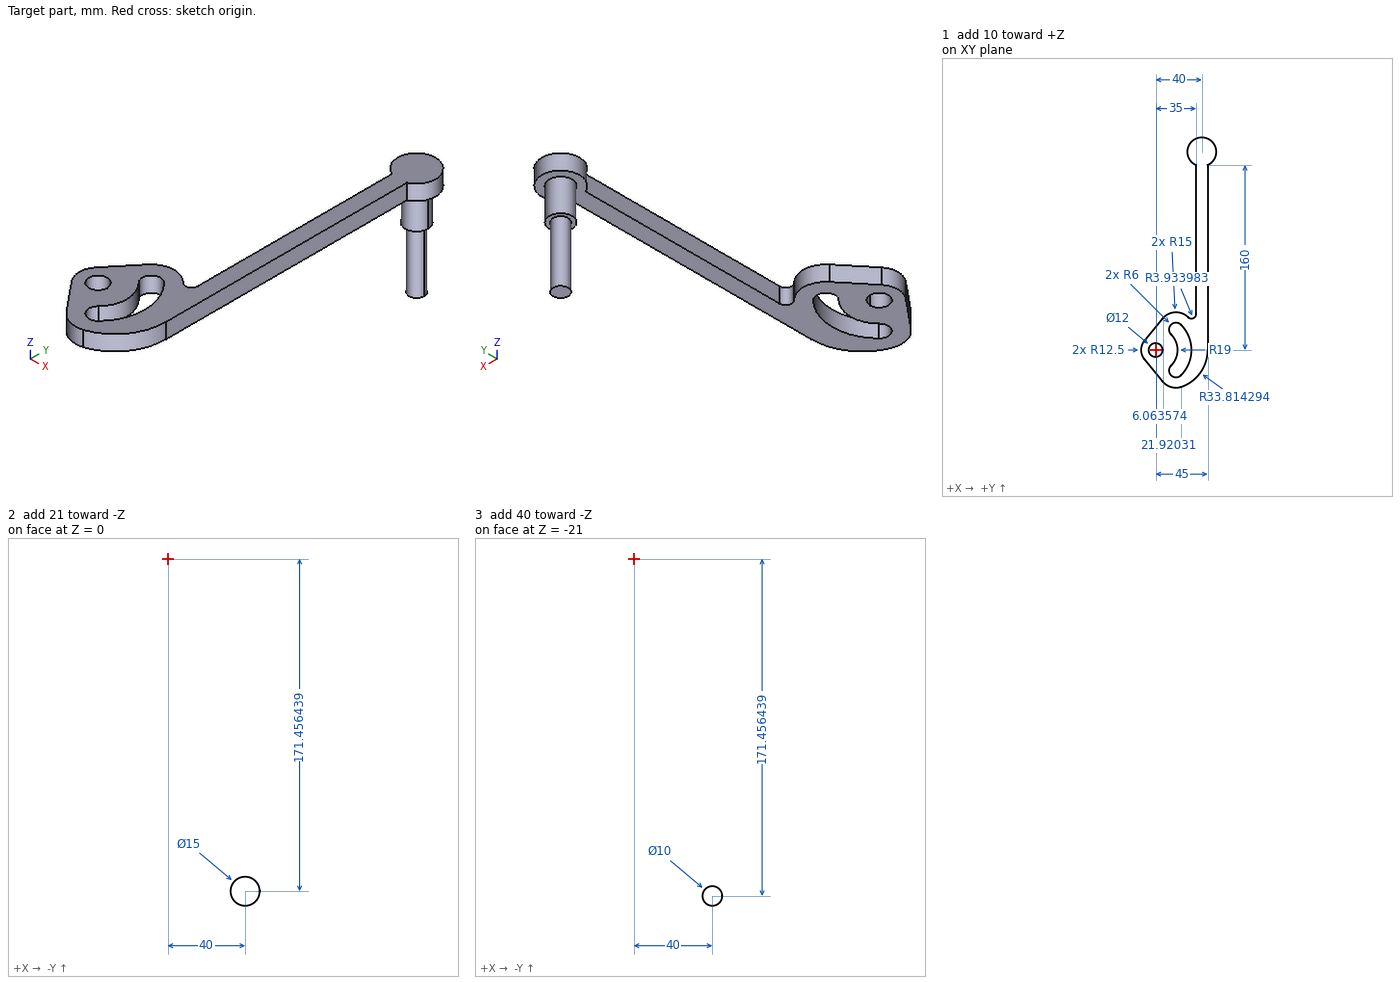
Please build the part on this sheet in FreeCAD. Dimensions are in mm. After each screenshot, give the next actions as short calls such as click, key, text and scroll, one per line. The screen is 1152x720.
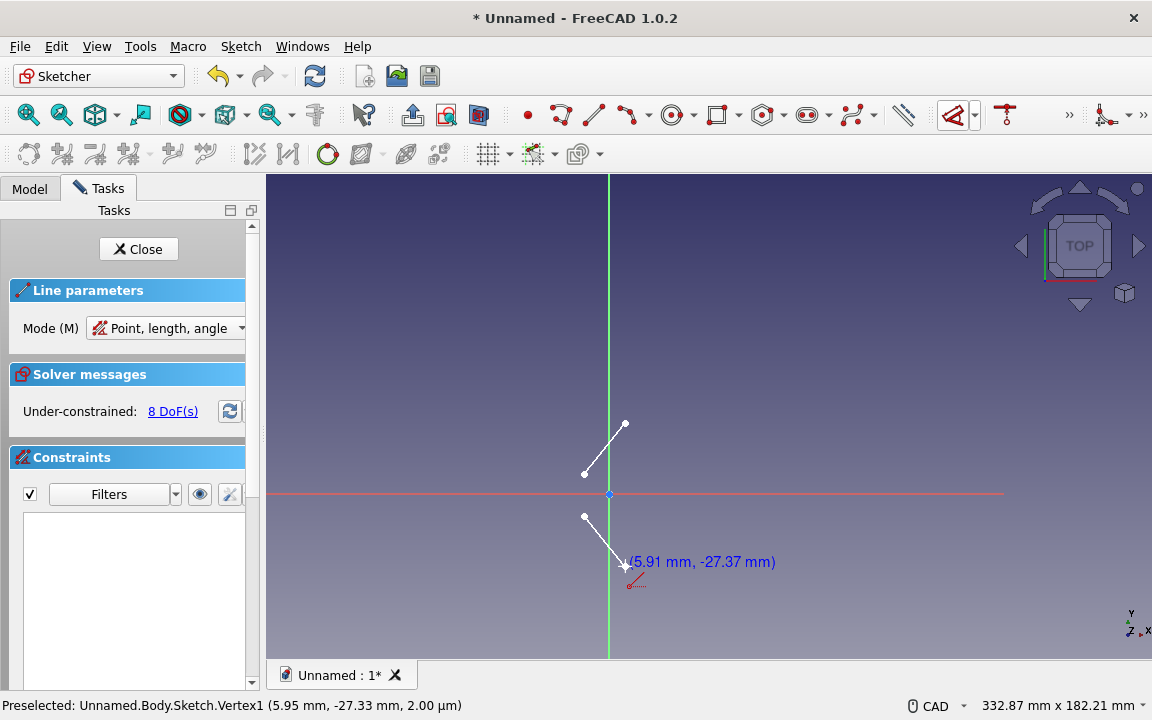
click(729, 494)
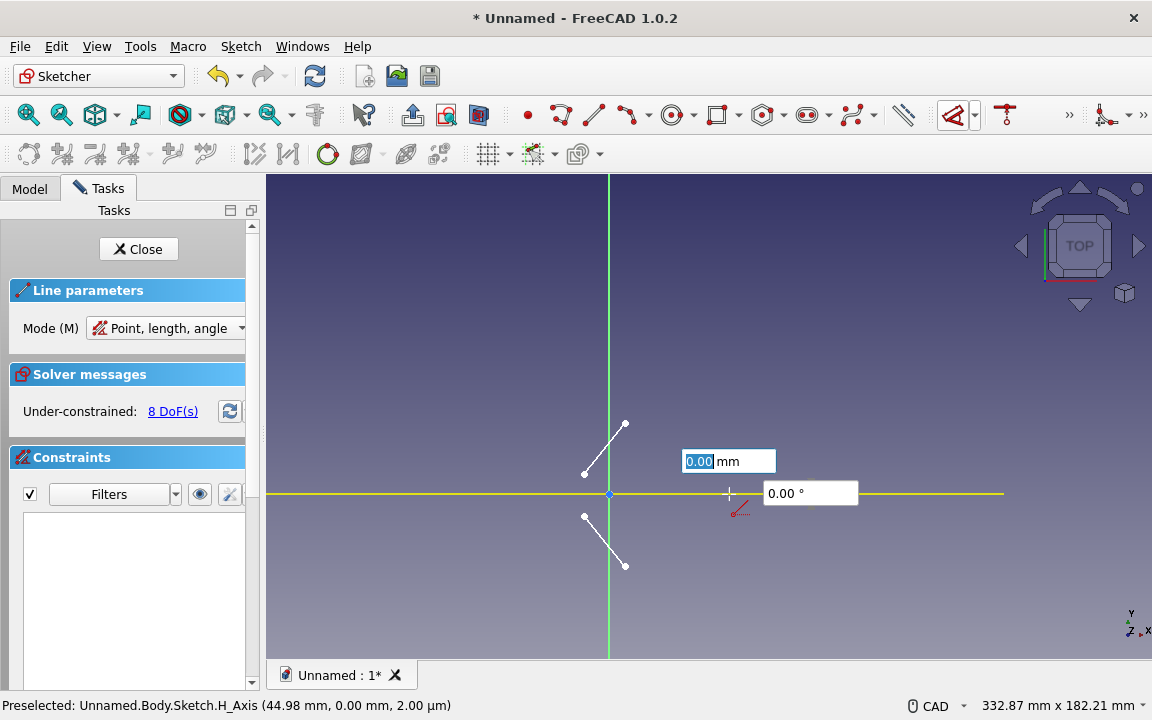
scroll(626, 568, down, 3)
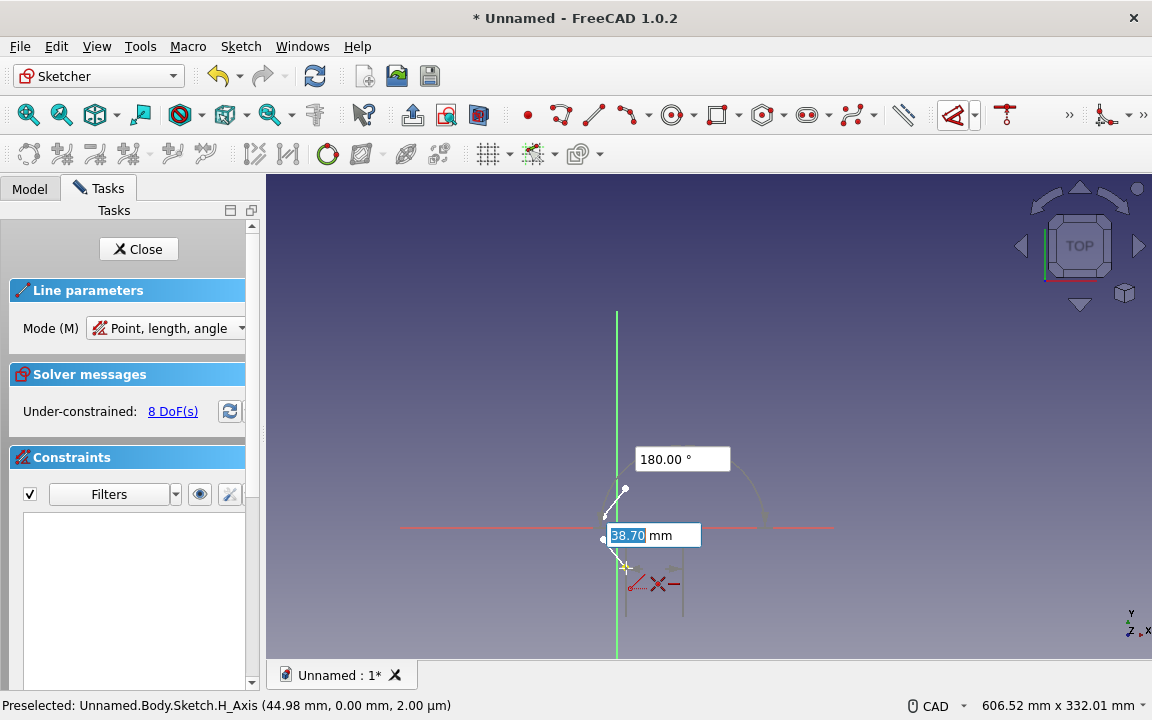
click(683, 294)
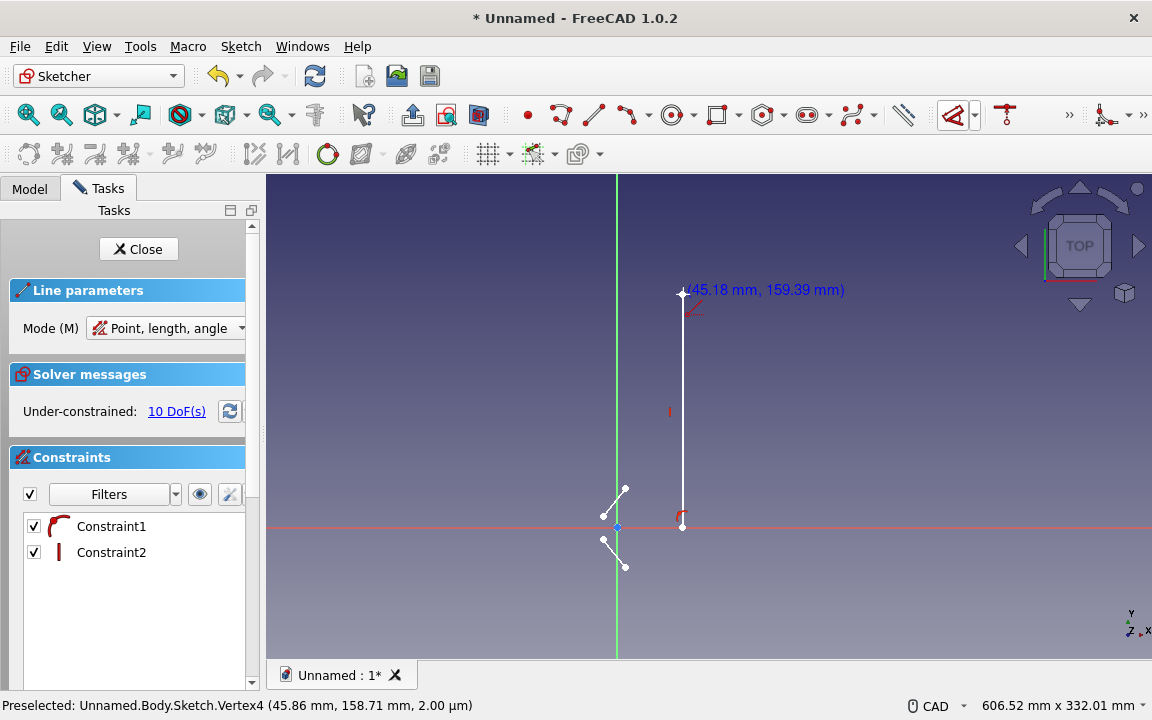
click(668, 294)
click(668, 482)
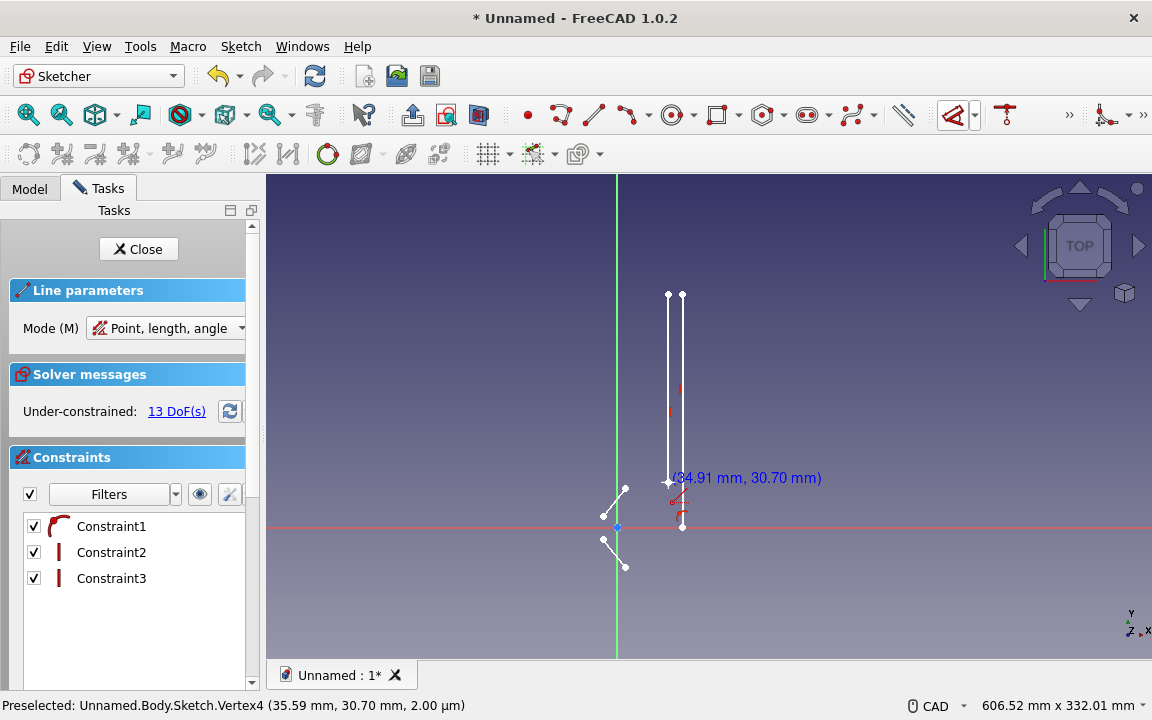
key(g)
key(3)
key(a)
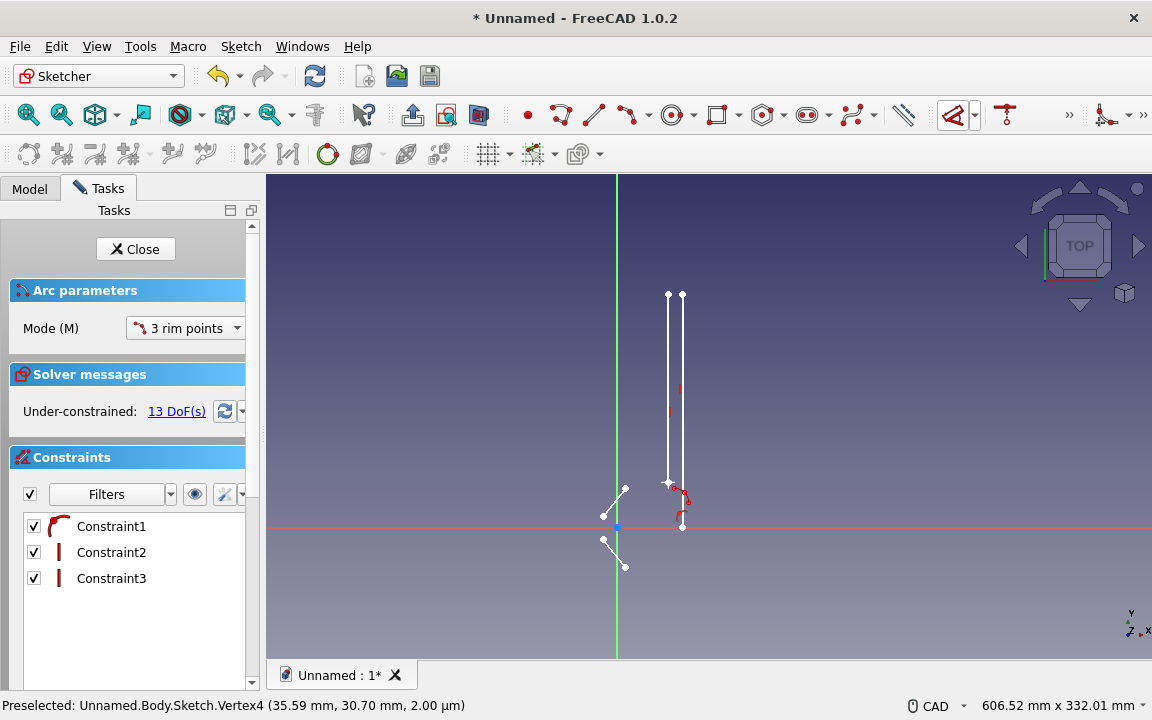
scroll(603, 516, up, 2)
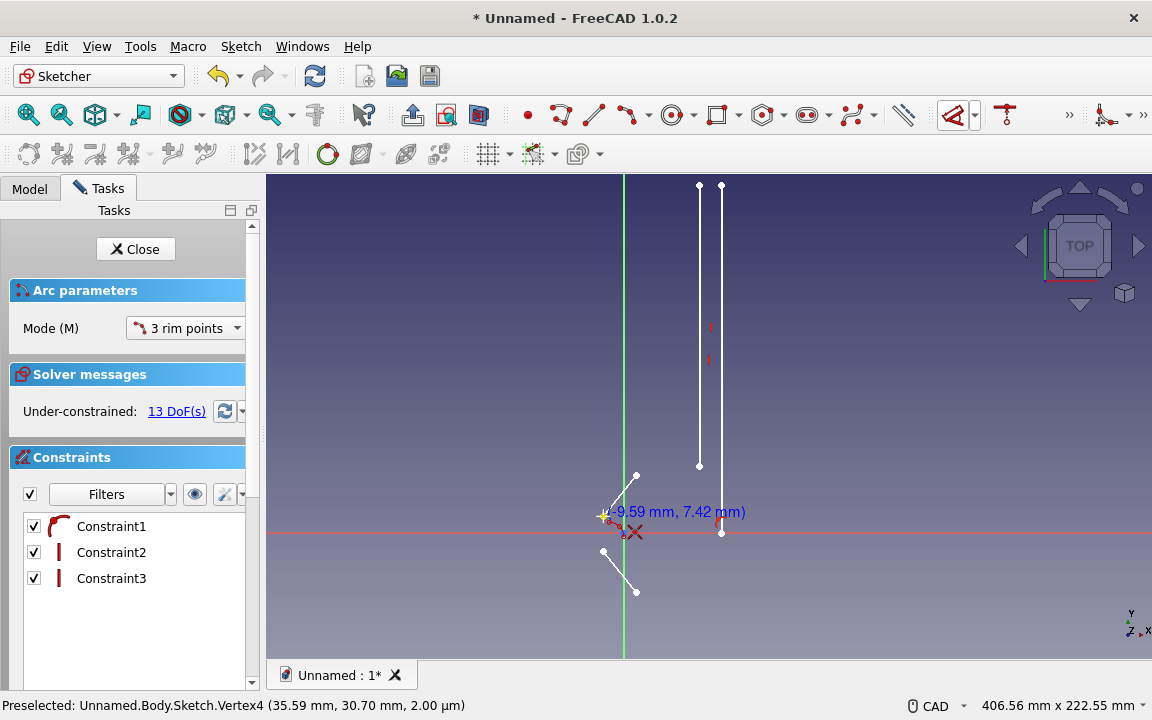
click(603, 517)
click(603, 551)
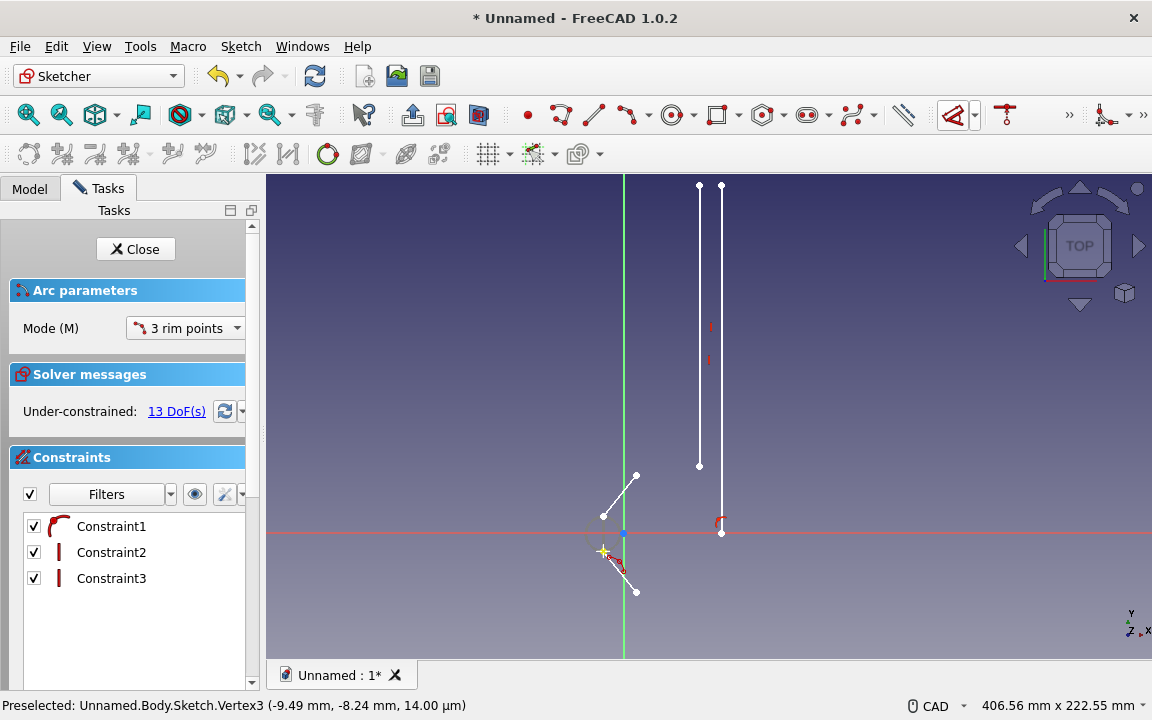
scroll(597, 526, up, 6)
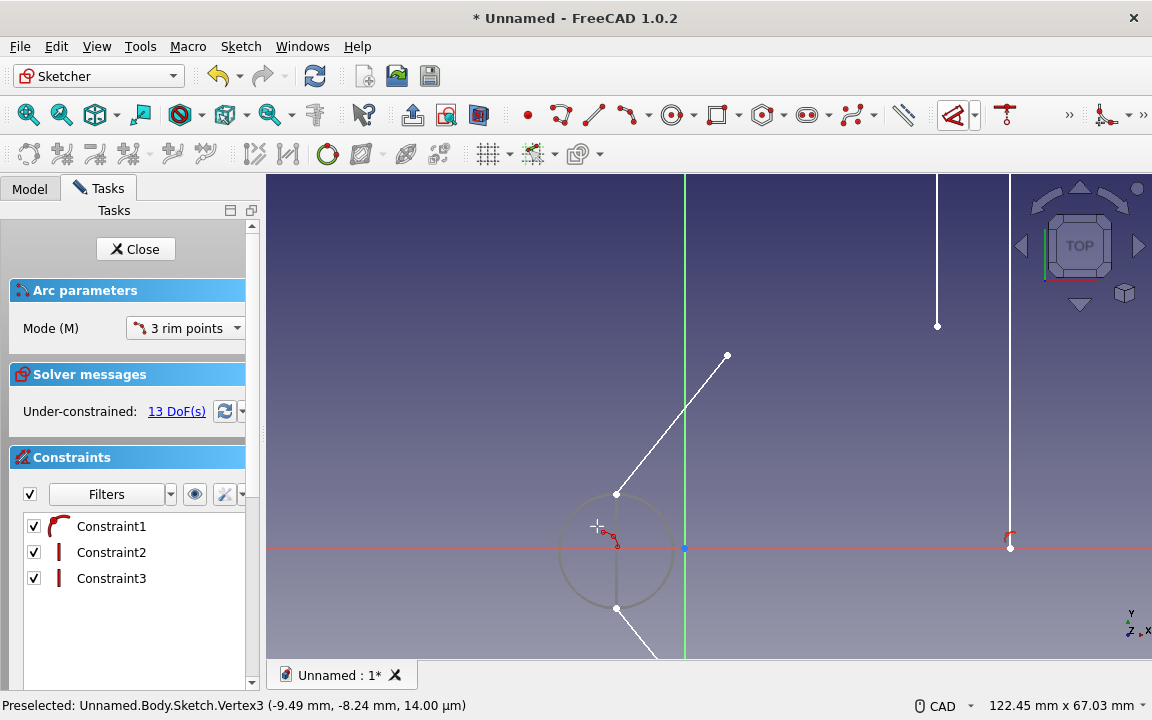
click(598, 524)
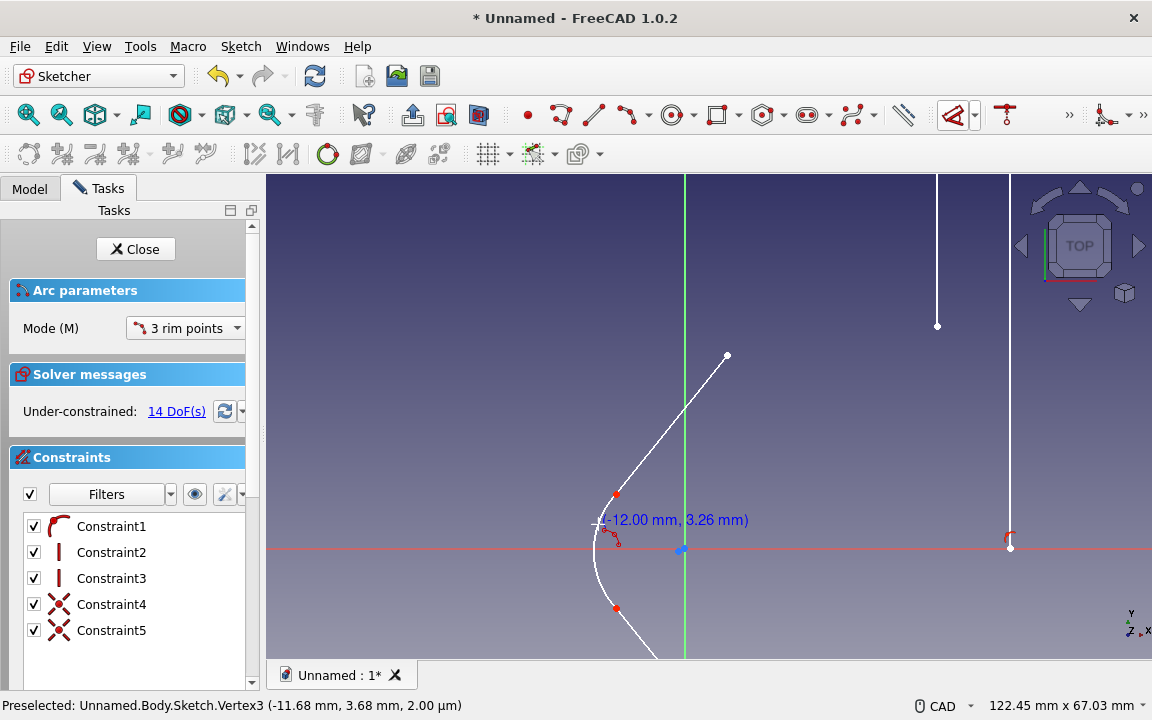
scroll(600, 522, down, 8)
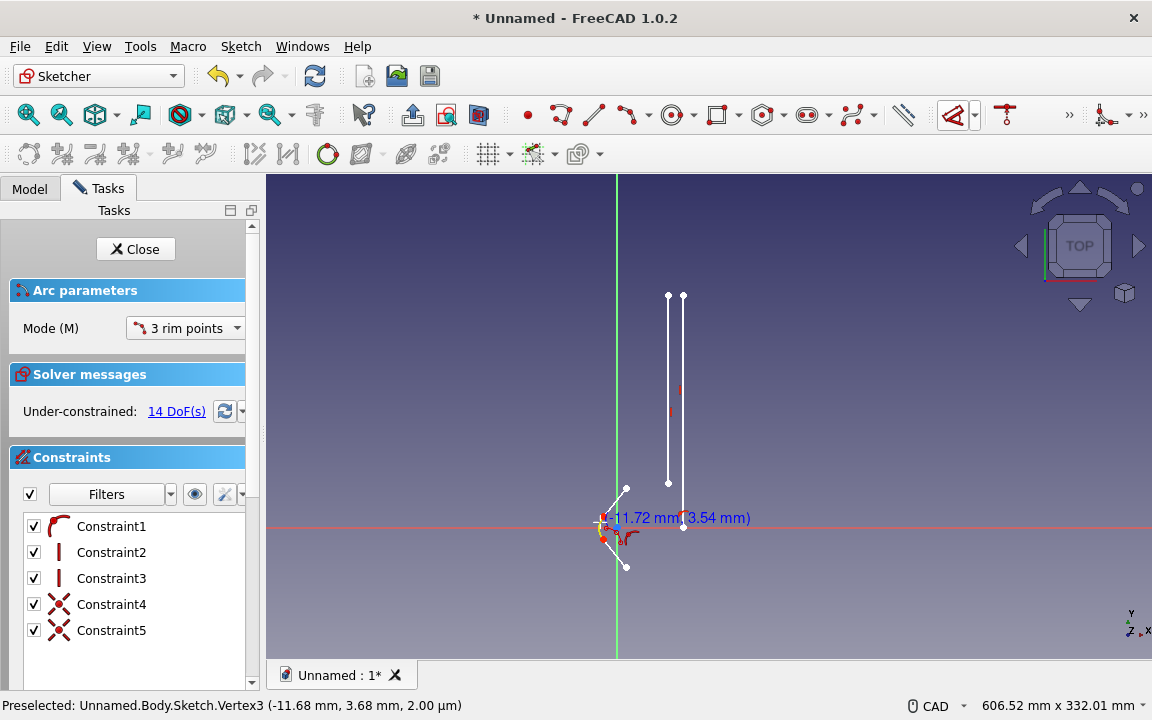
scroll(626, 568, up, 3)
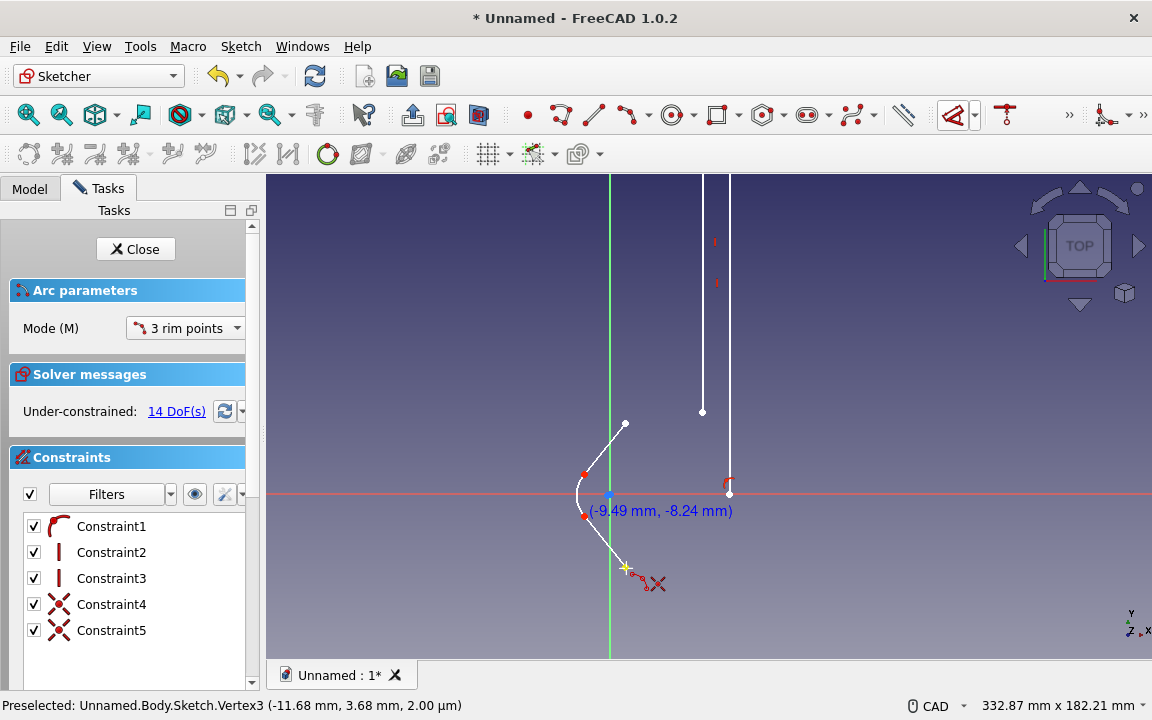
click(626, 567)
click(668, 580)